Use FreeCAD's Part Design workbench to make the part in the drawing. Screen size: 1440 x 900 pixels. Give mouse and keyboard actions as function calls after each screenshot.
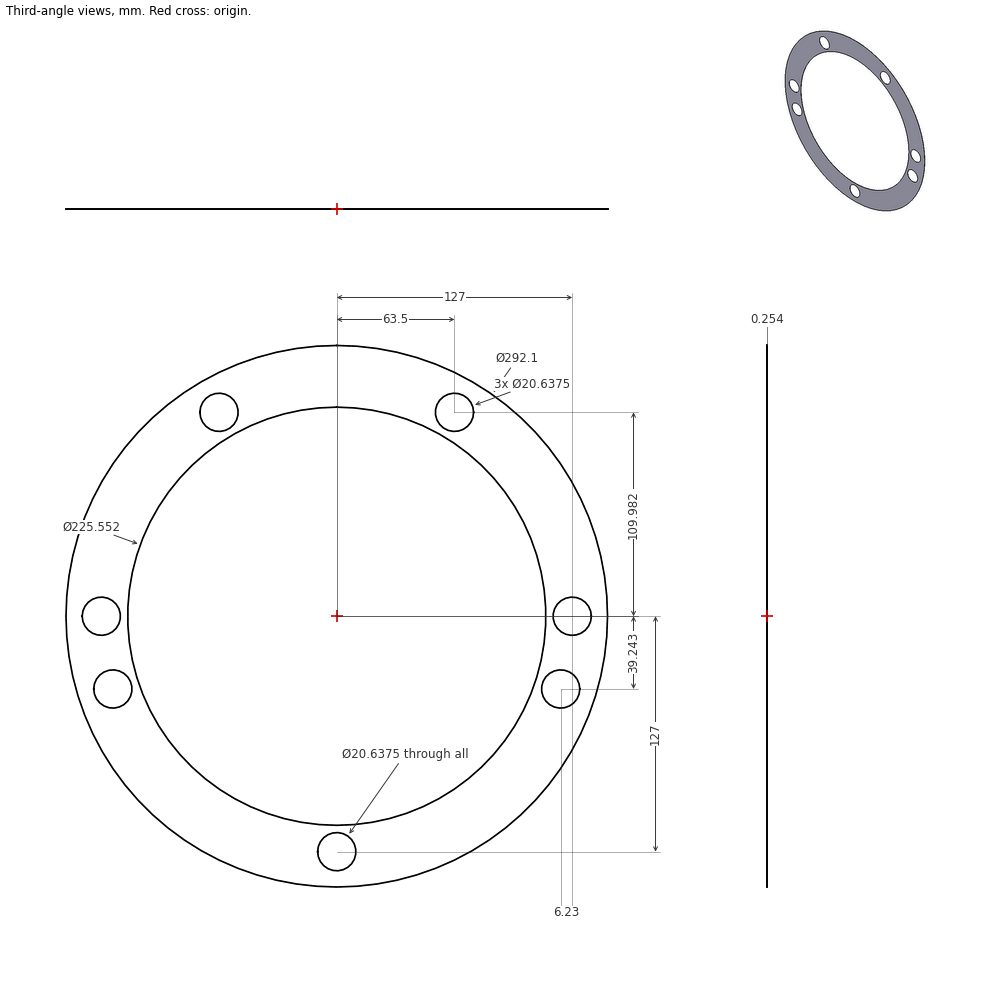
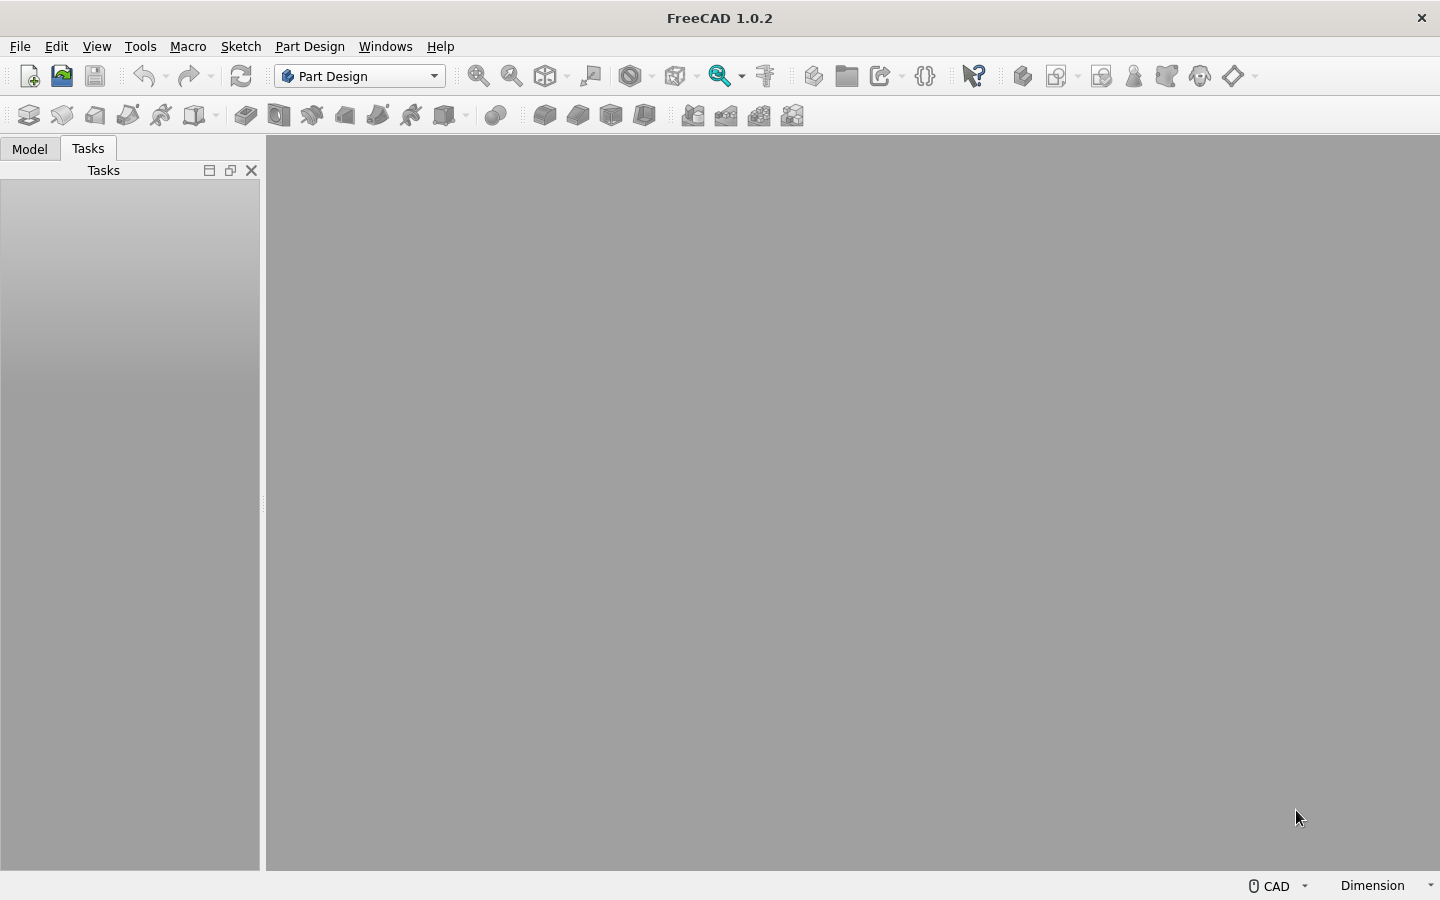
click(29, 76)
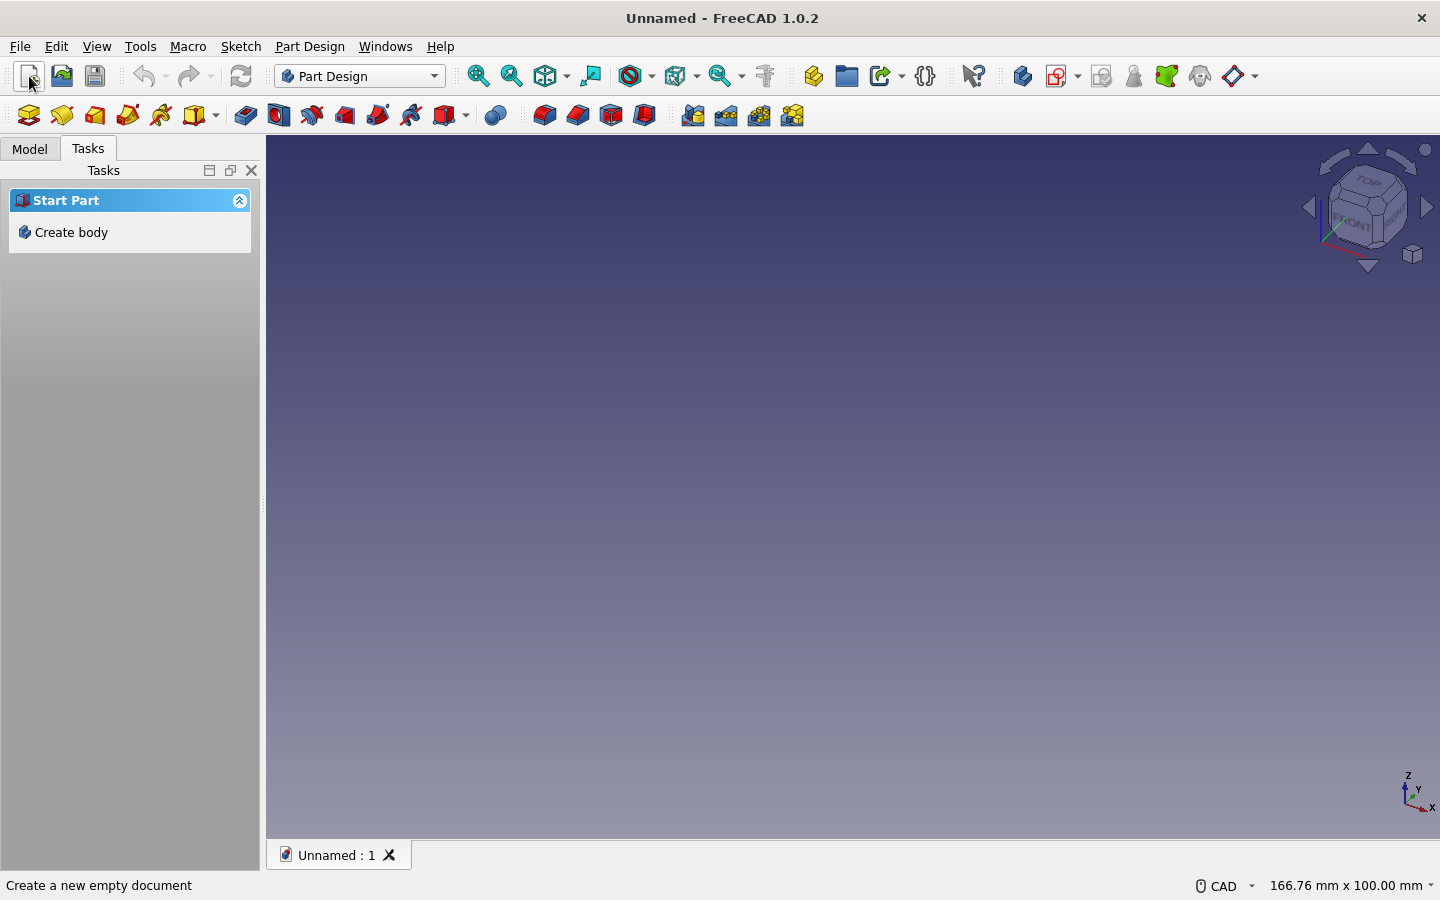
click(1056, 76)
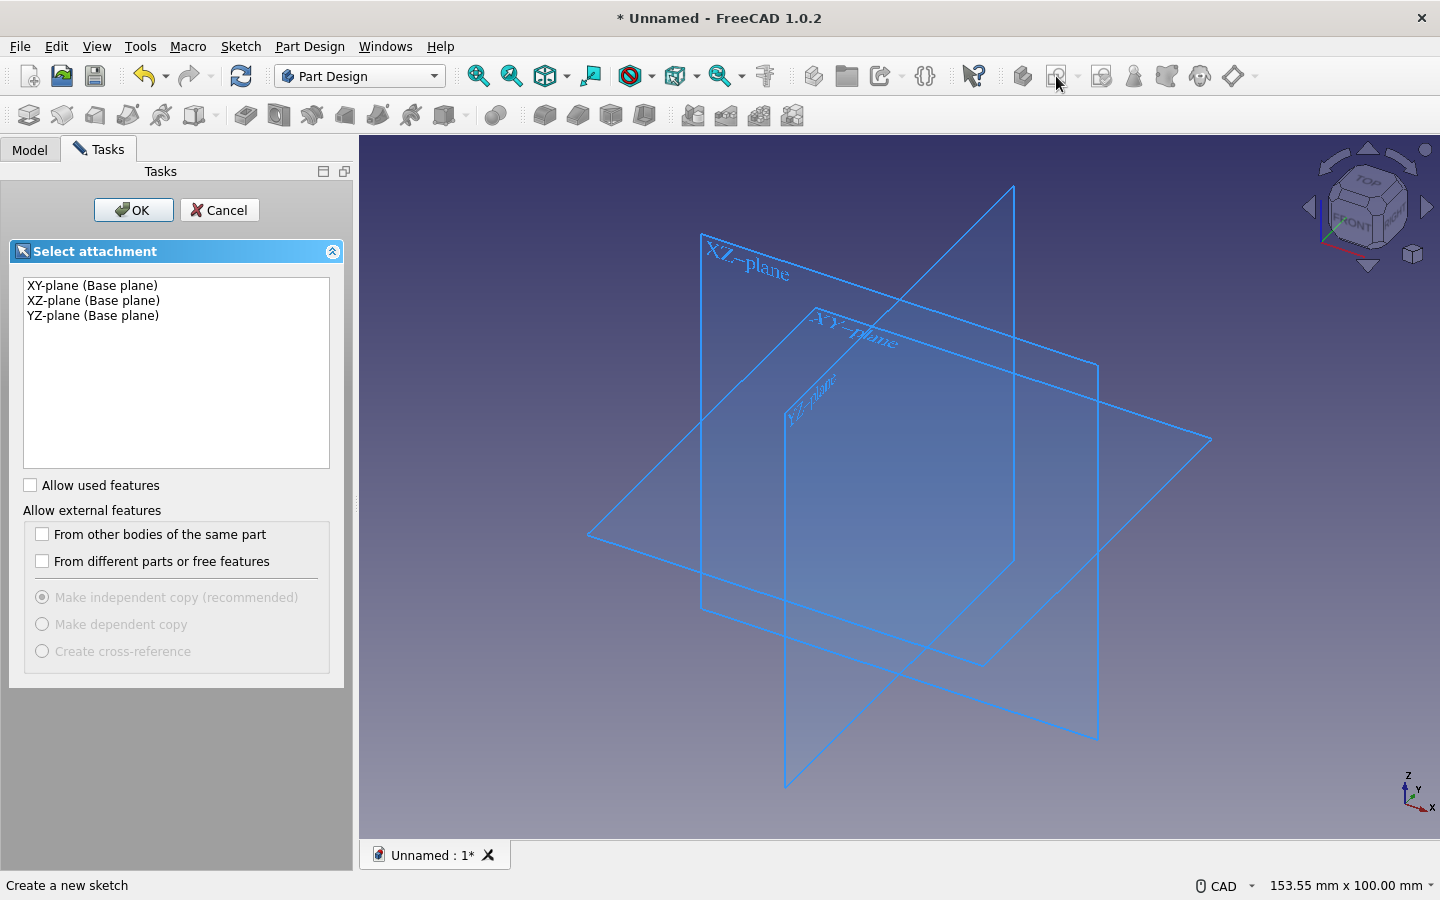
click(84, 300)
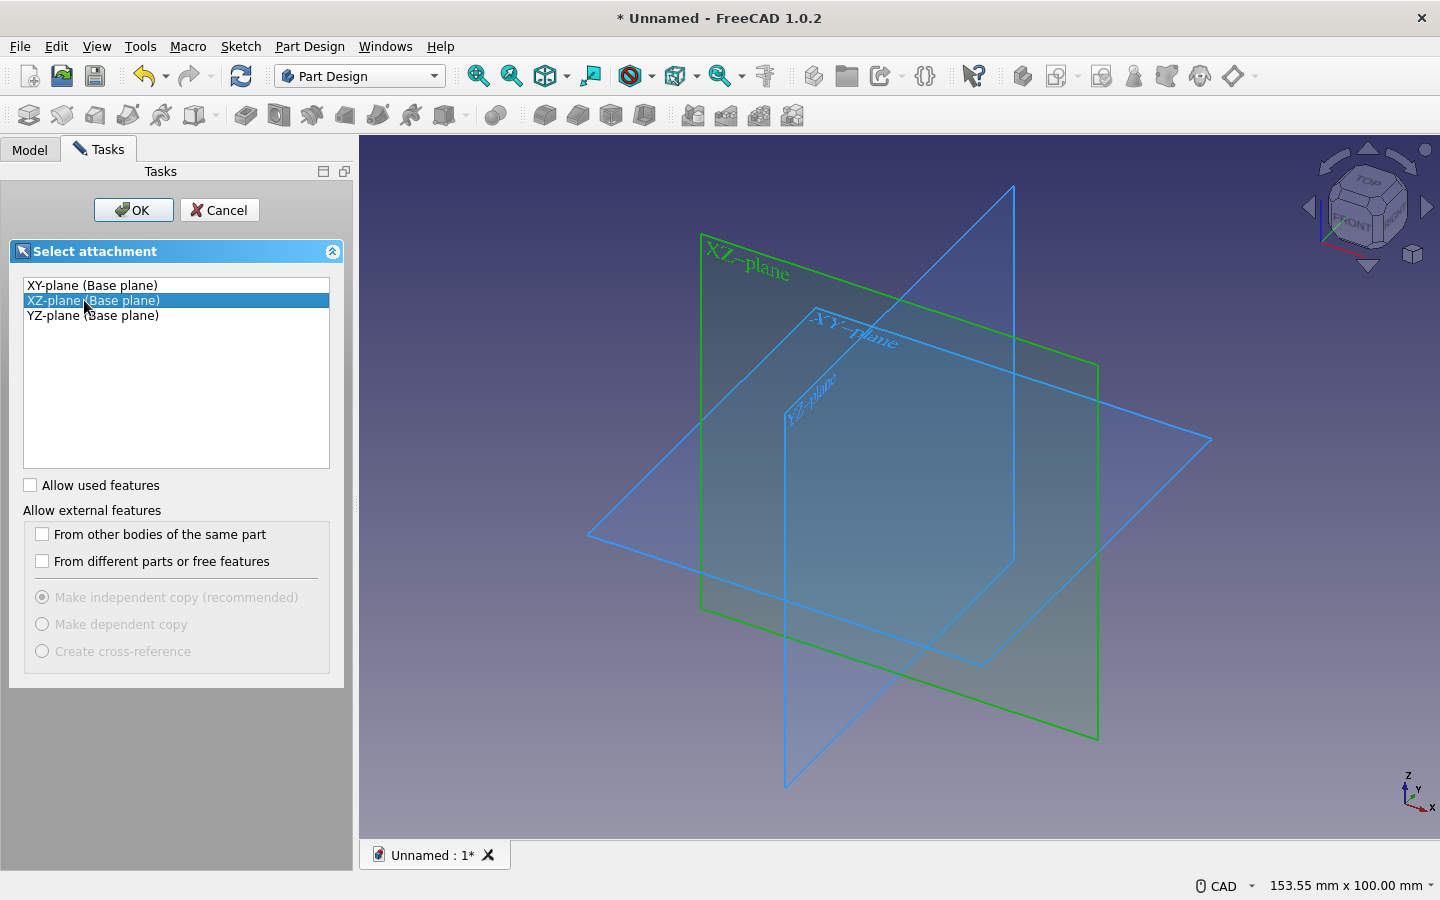
click(134, 210)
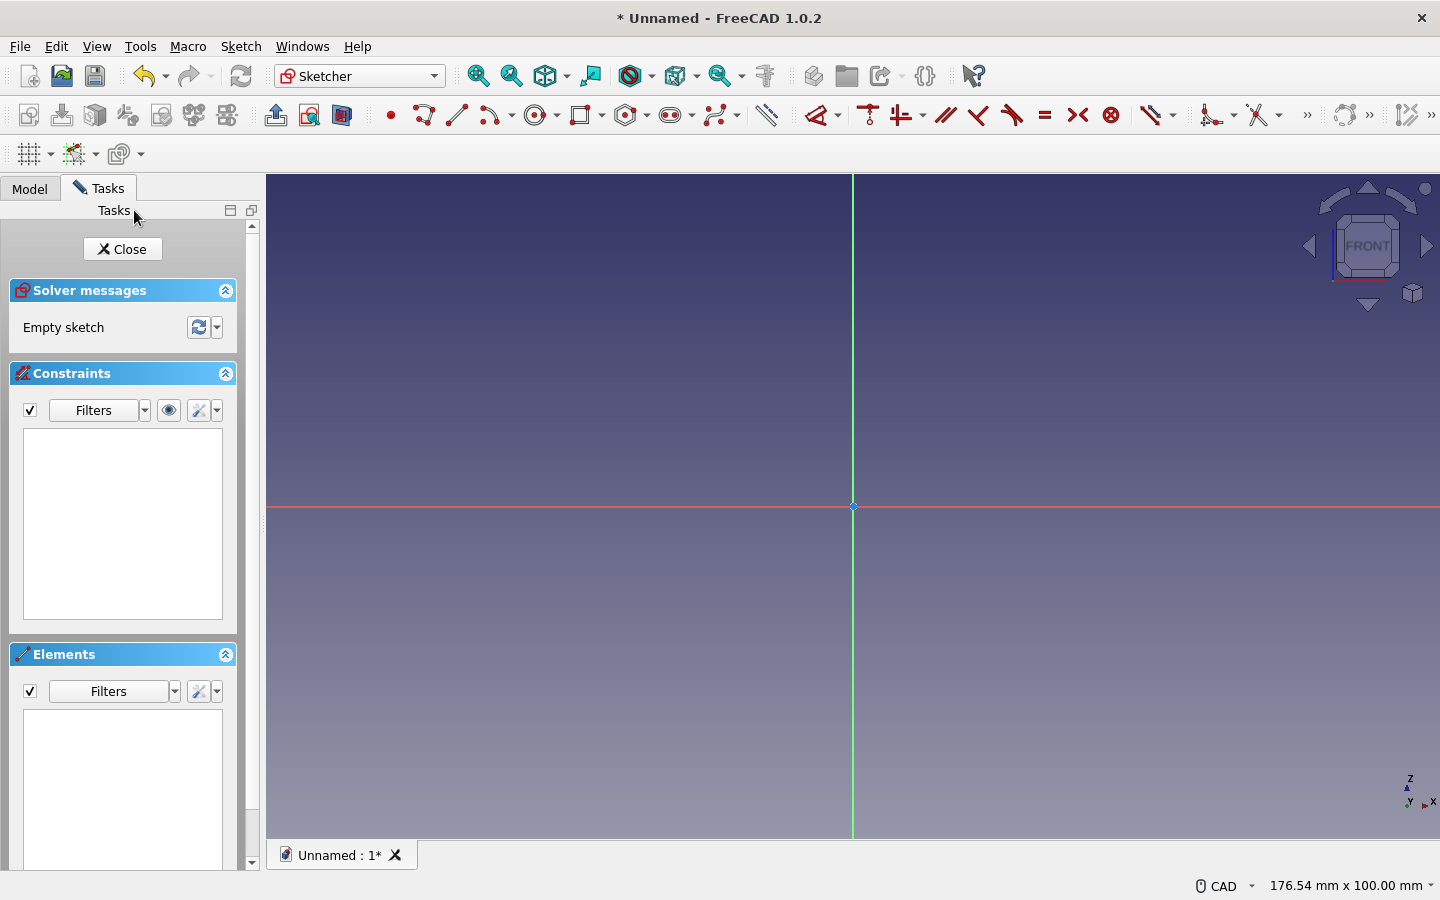
scroll(767, 506, down, 8)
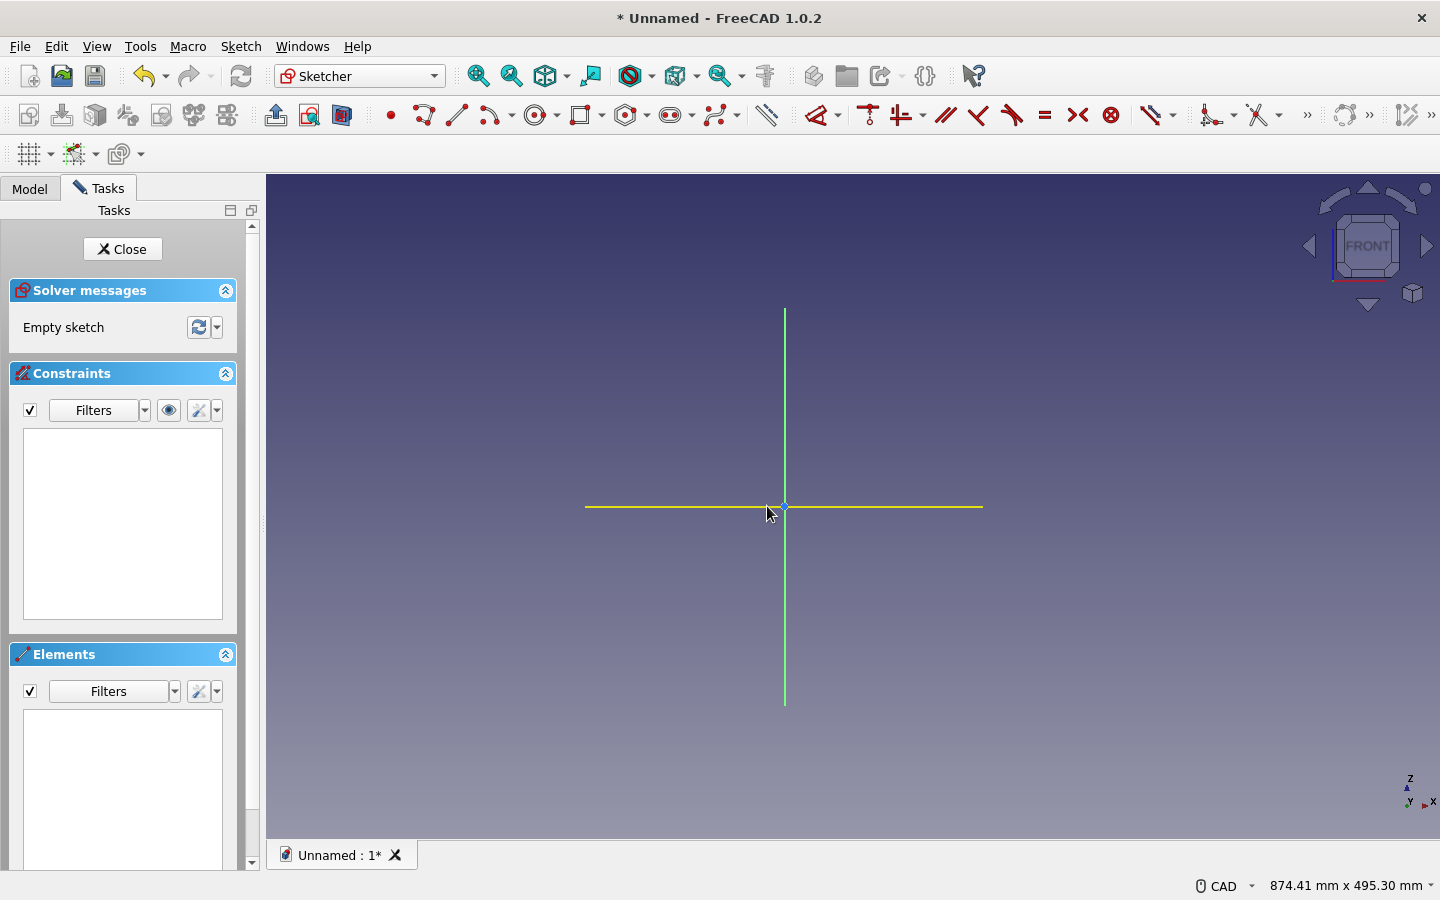
click(534, 116)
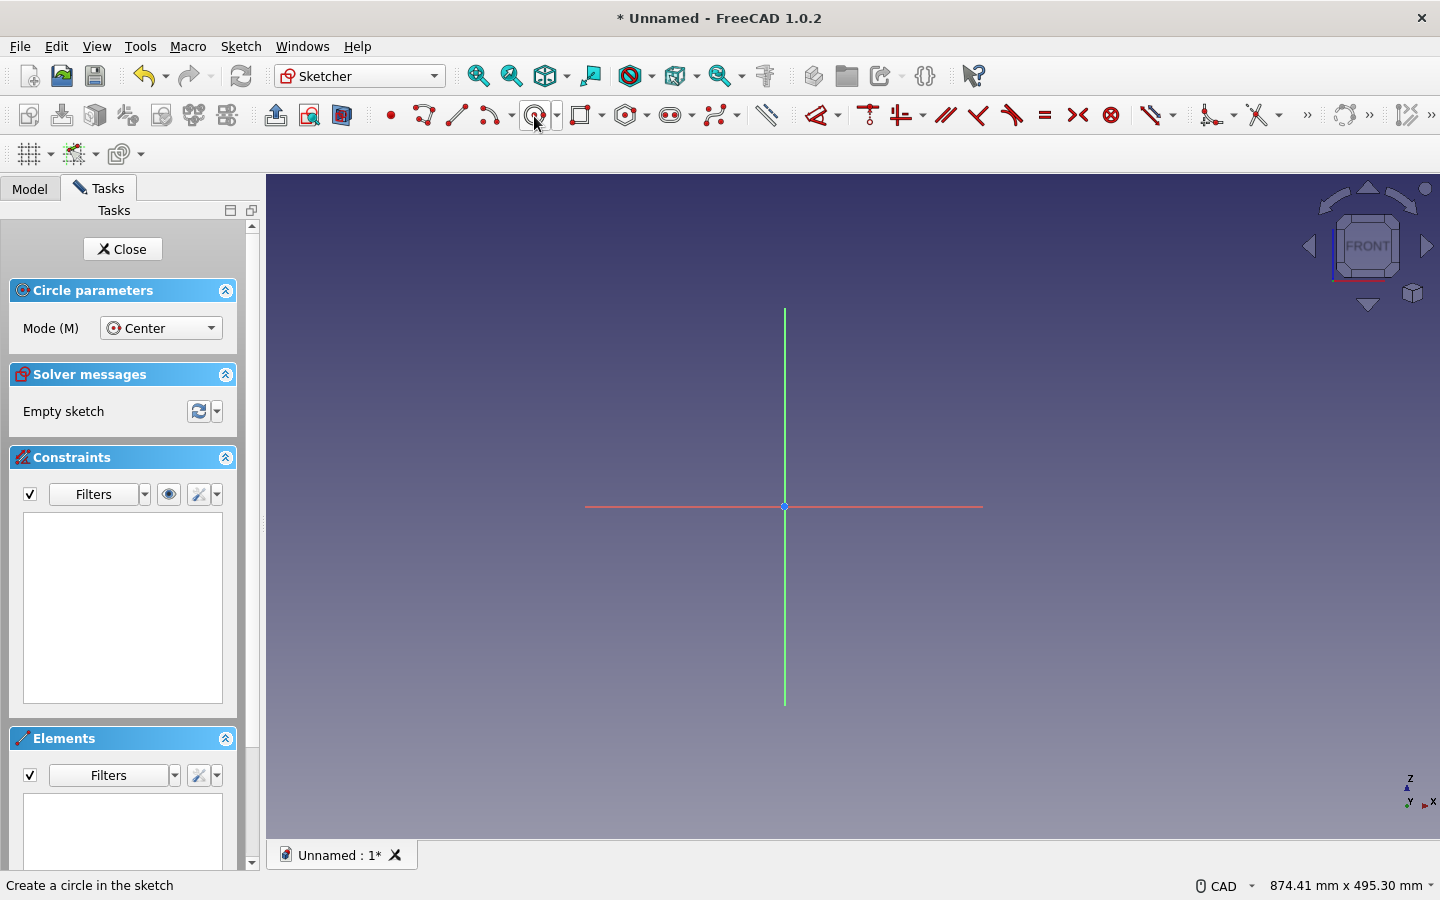
click(785, 506)
click(923, 368)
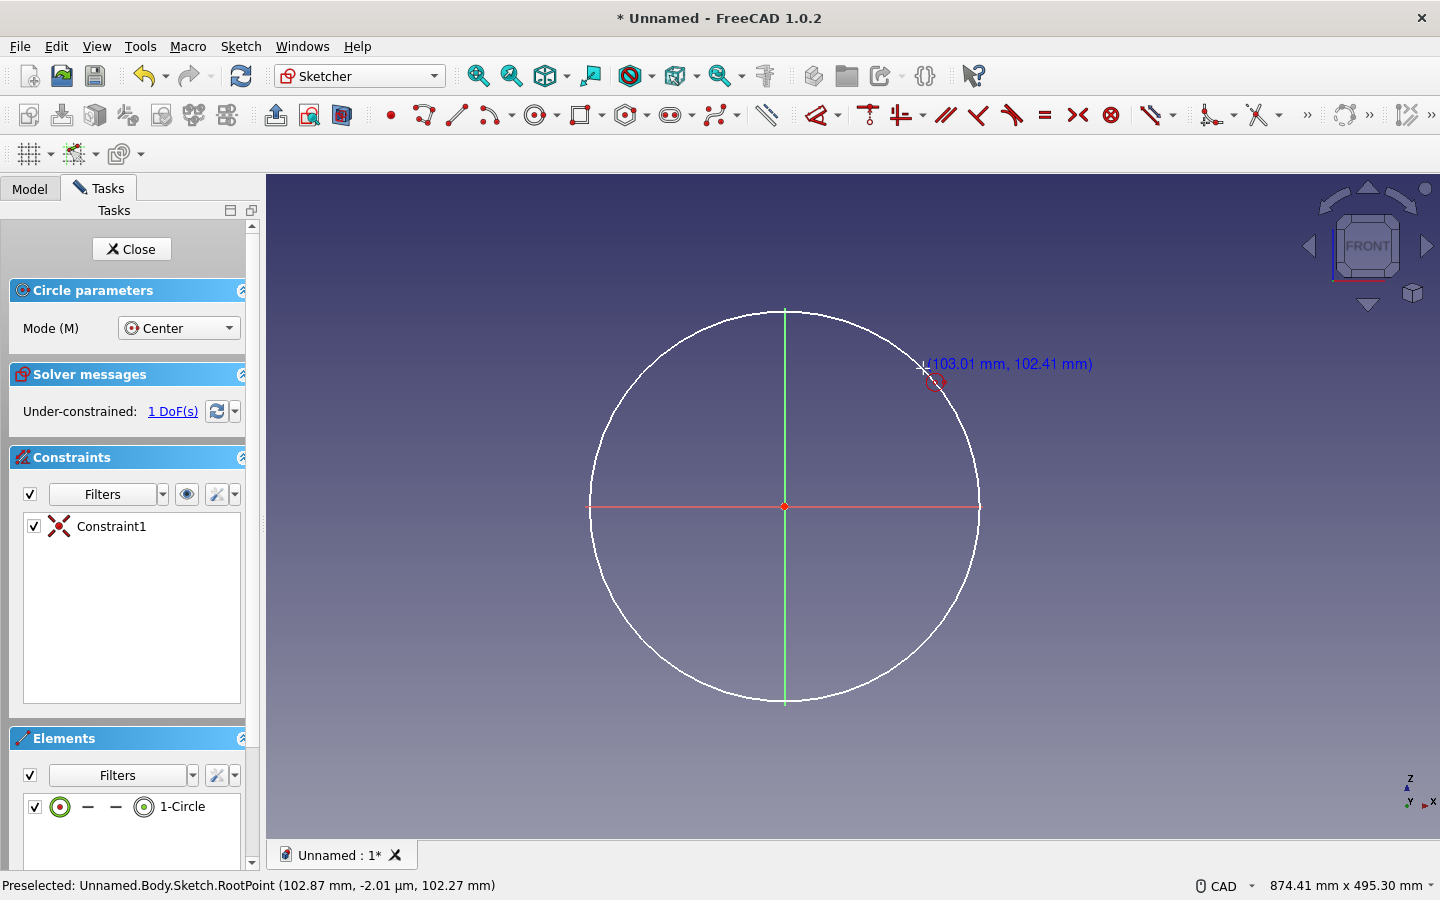
click(785, 506)
click(892, 399)
key(Escape)